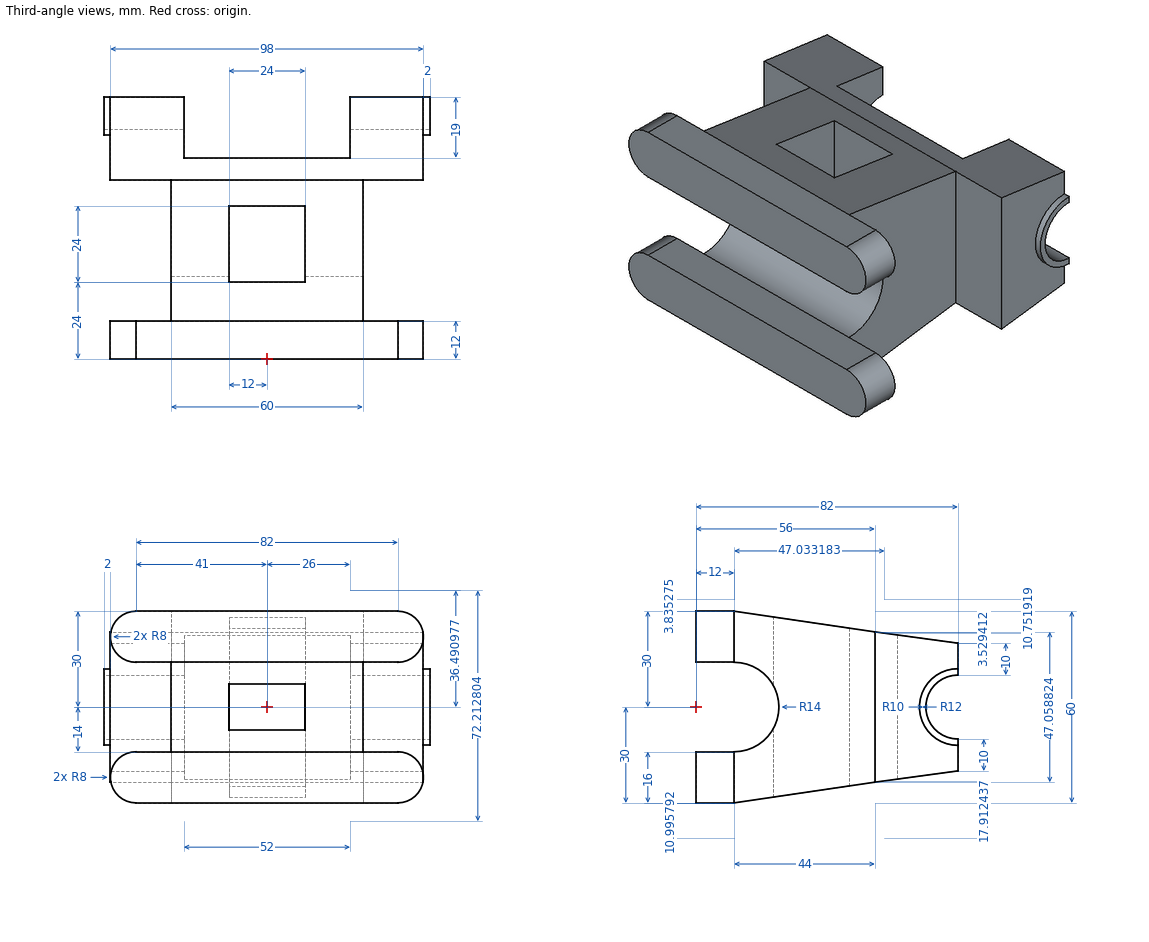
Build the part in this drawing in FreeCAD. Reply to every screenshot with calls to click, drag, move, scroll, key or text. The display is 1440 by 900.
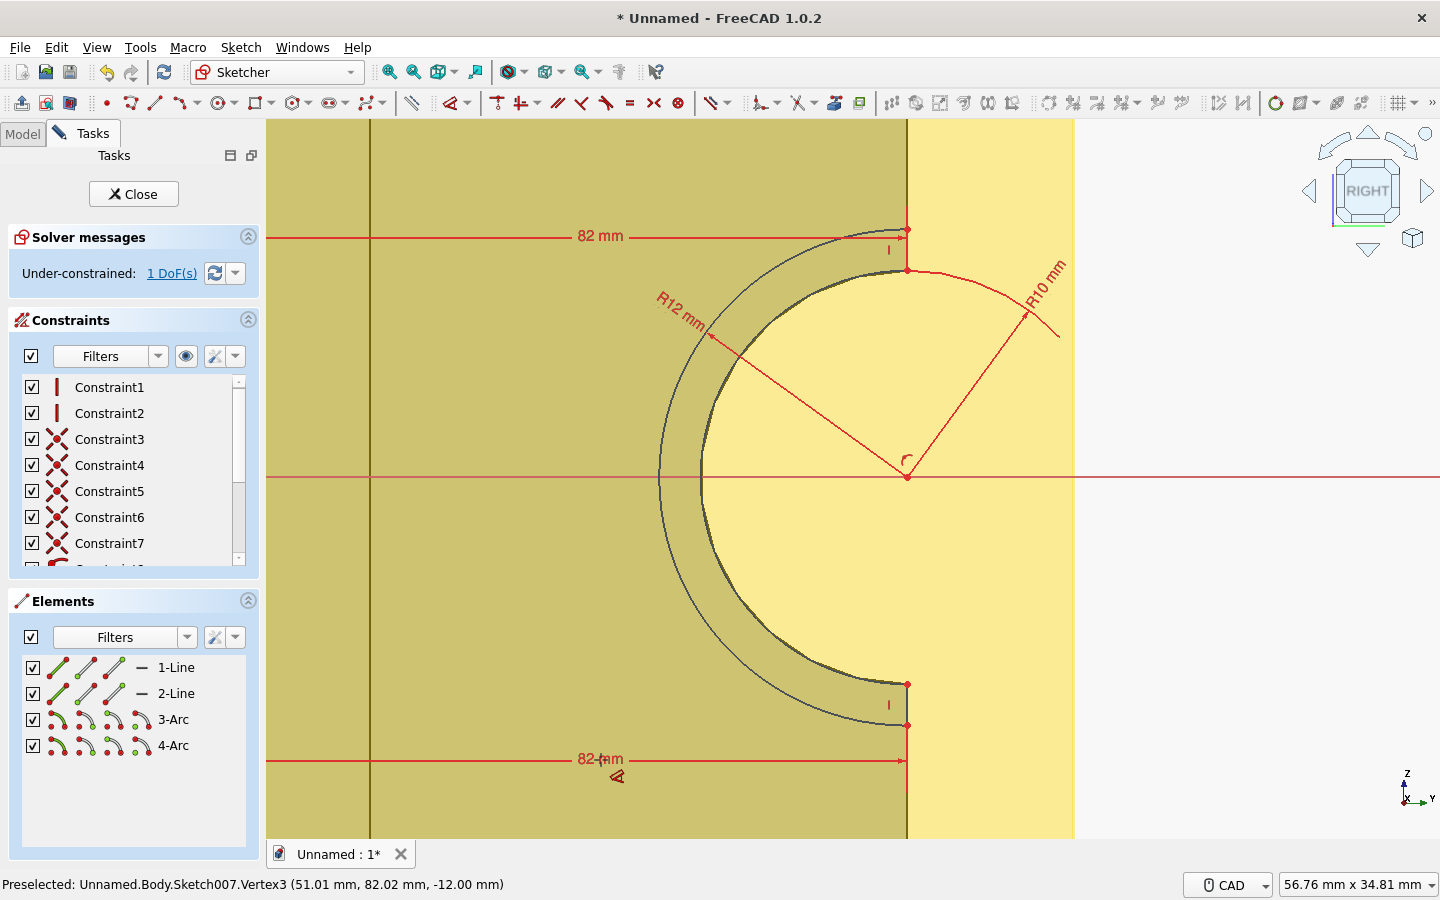
click(907, 477)
click(601, 511)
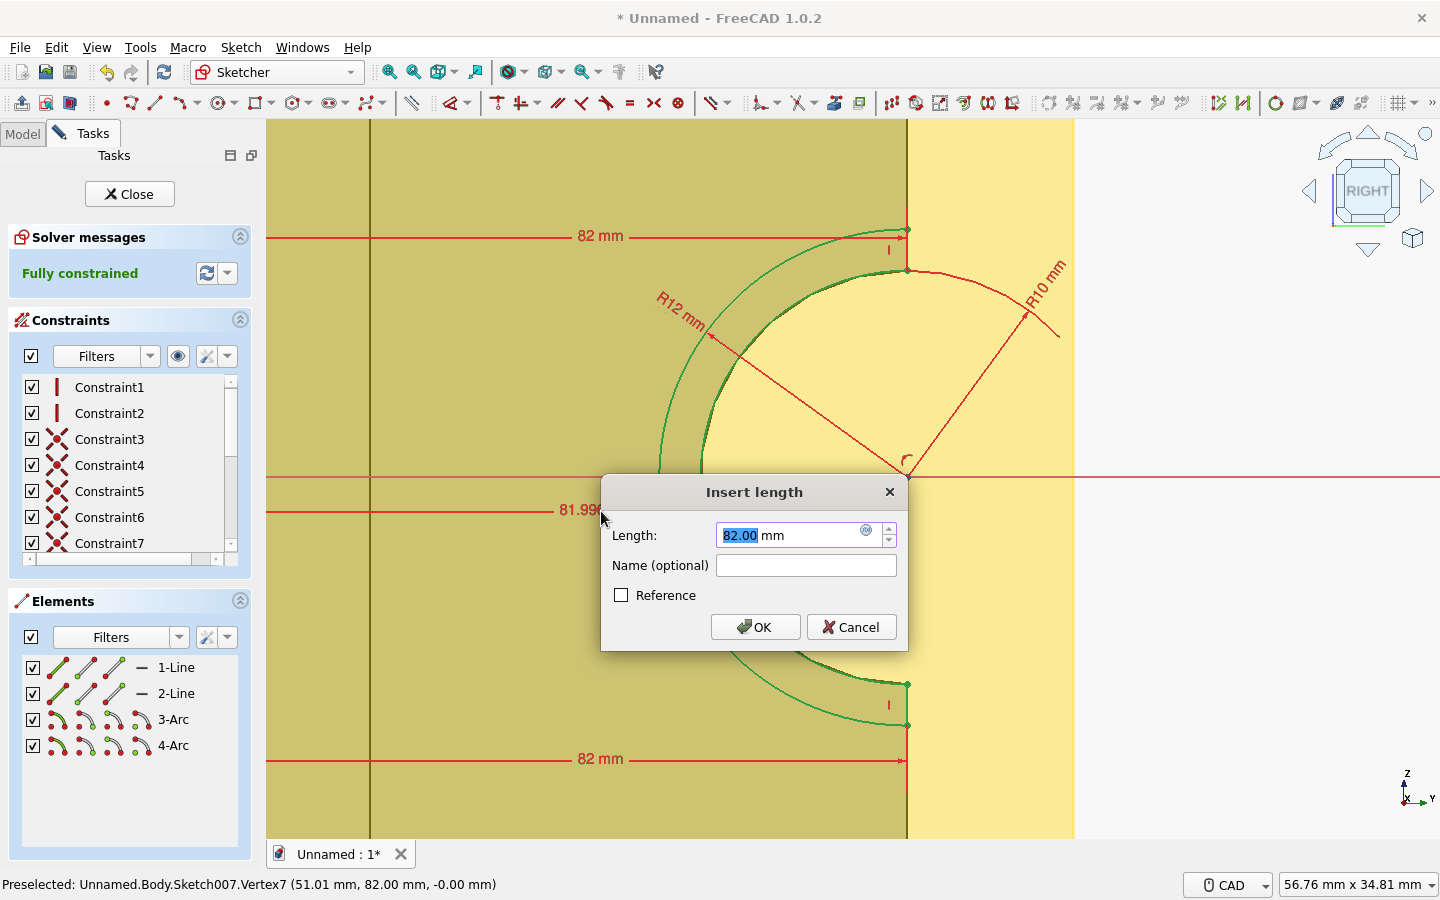
text(82)
key(Return)
key(Escape)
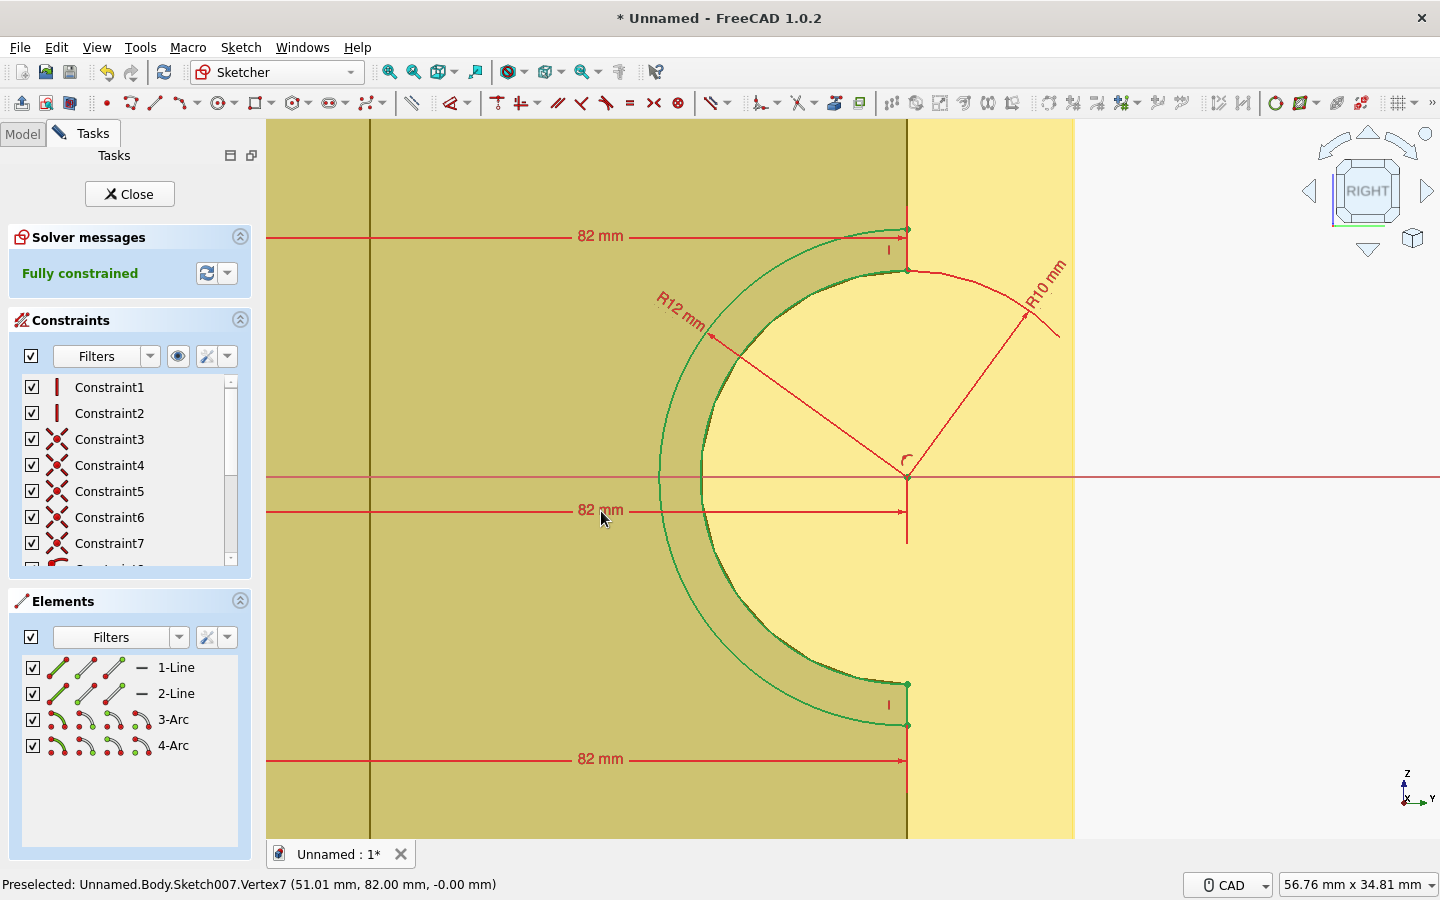
click(130, 194)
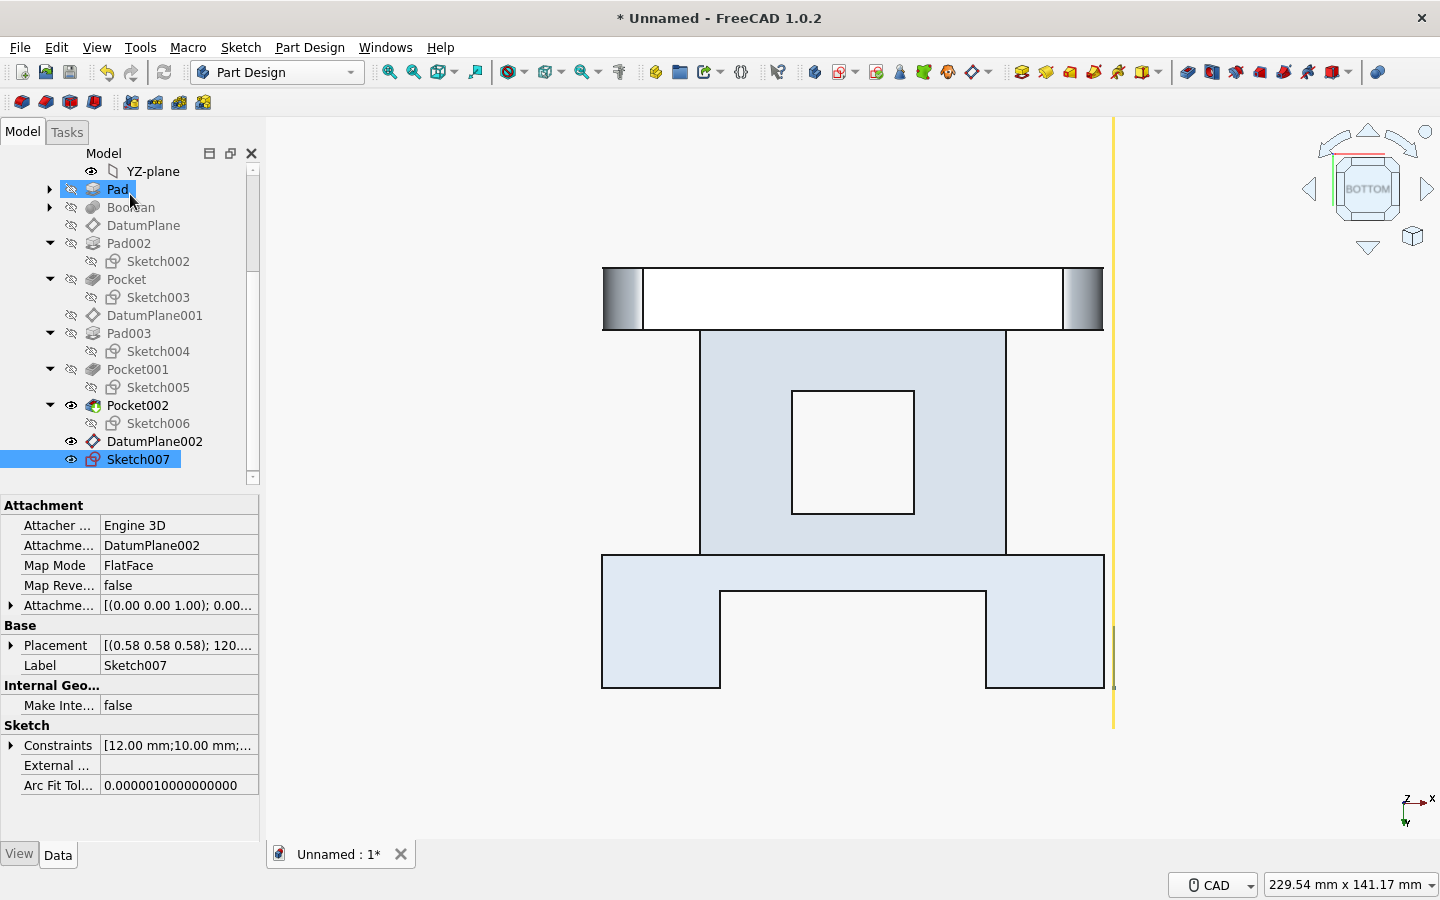
click(1022, 72)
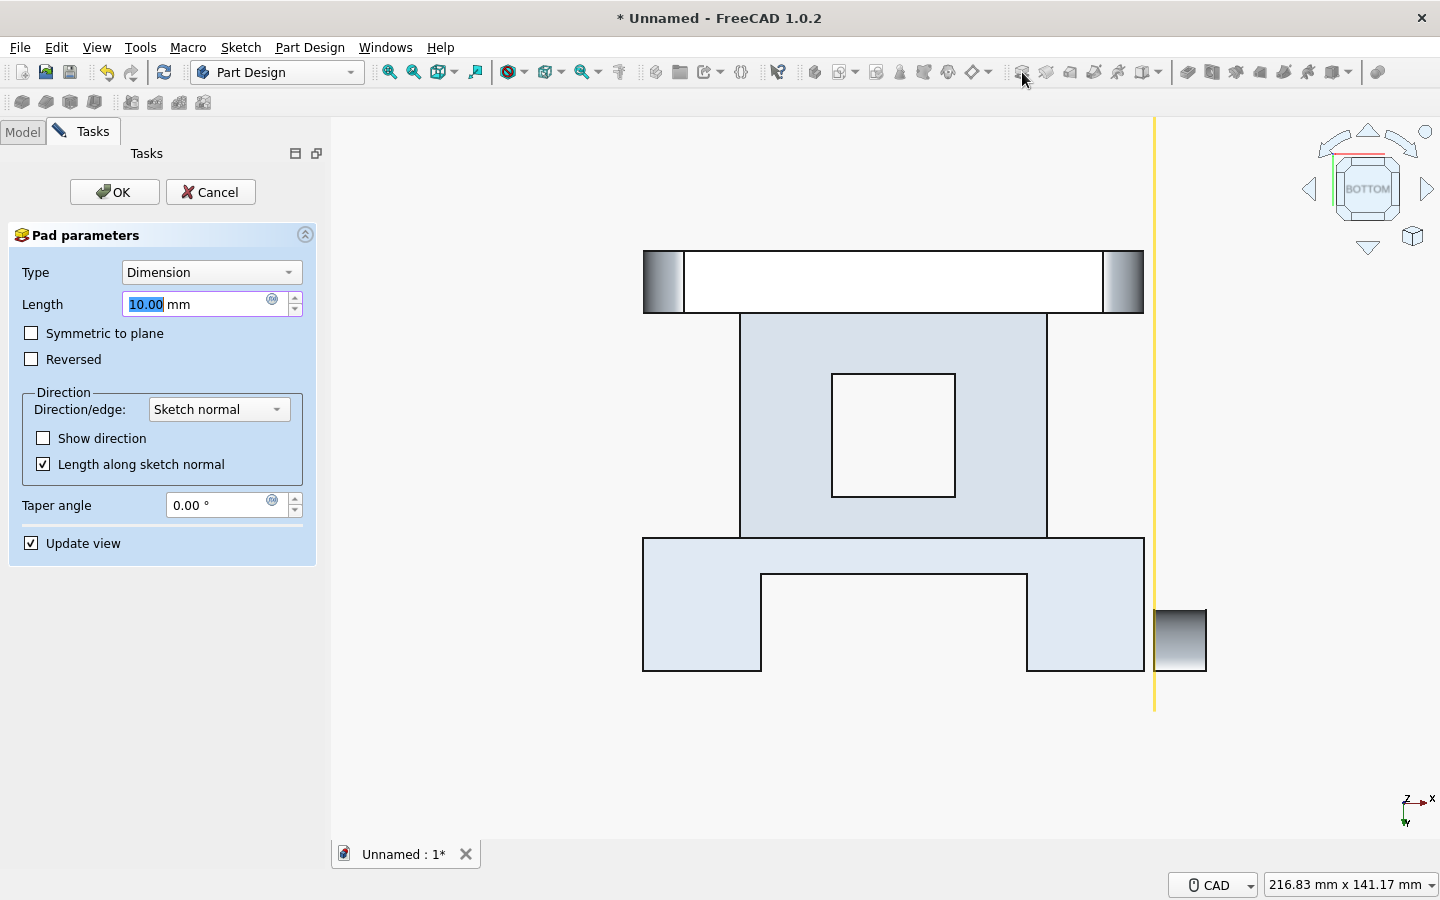
text(2)
key(Tab)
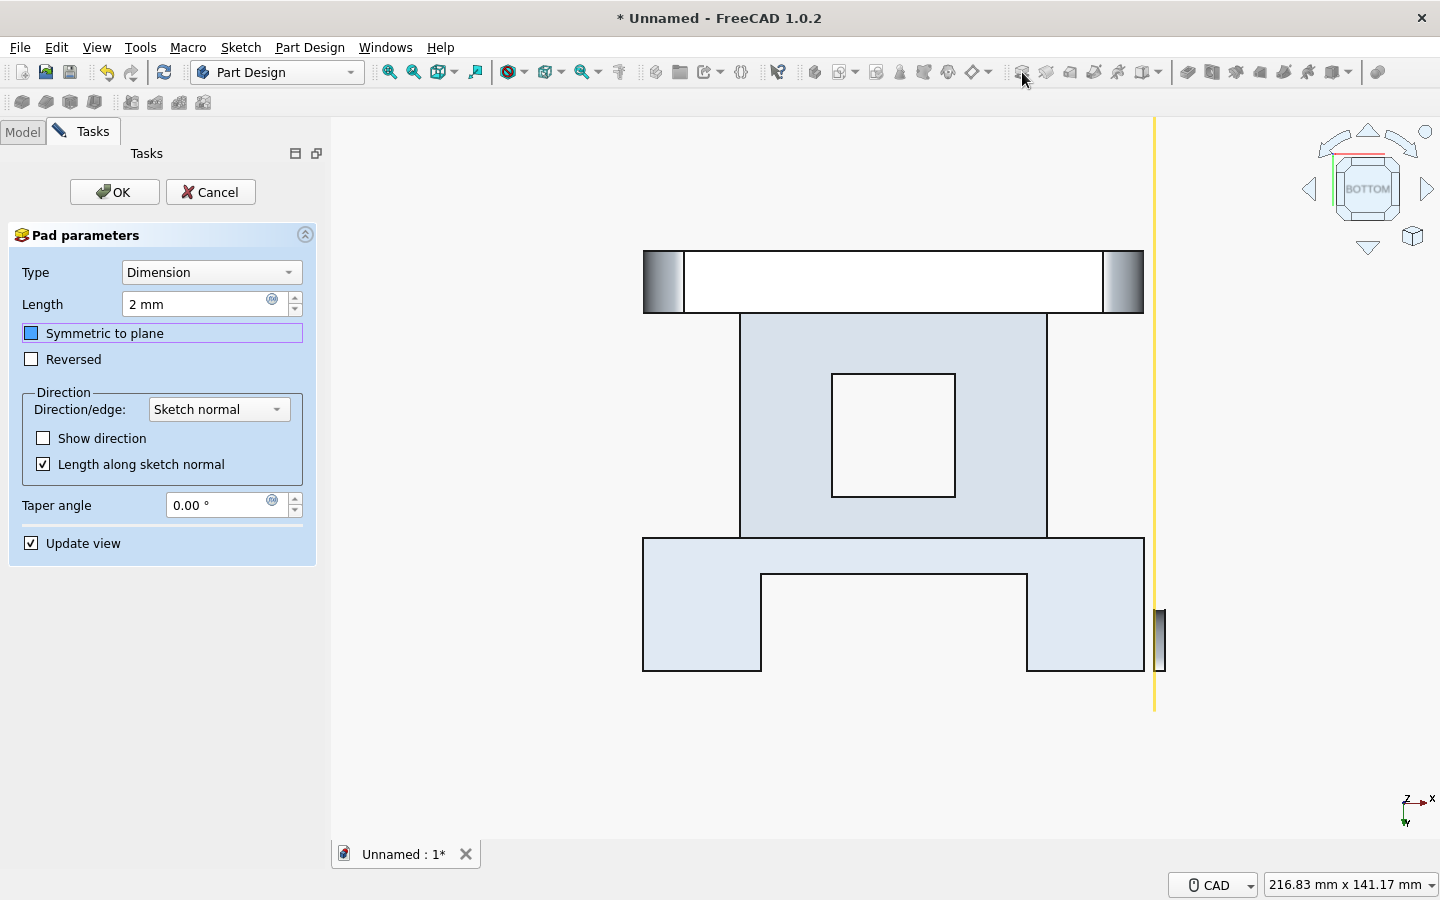
click(30, 359)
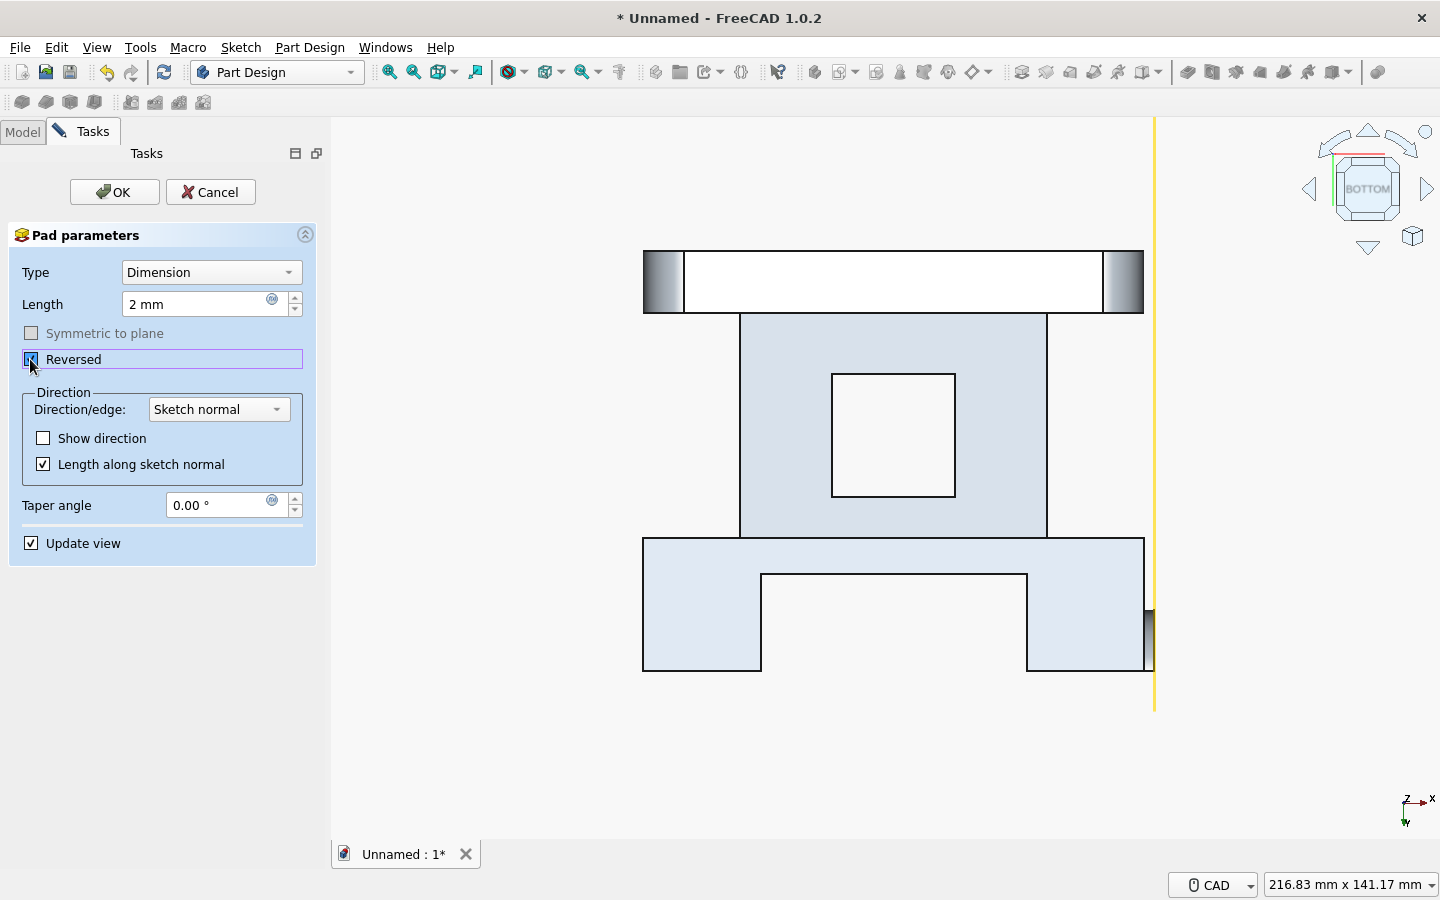
click(115, 192)